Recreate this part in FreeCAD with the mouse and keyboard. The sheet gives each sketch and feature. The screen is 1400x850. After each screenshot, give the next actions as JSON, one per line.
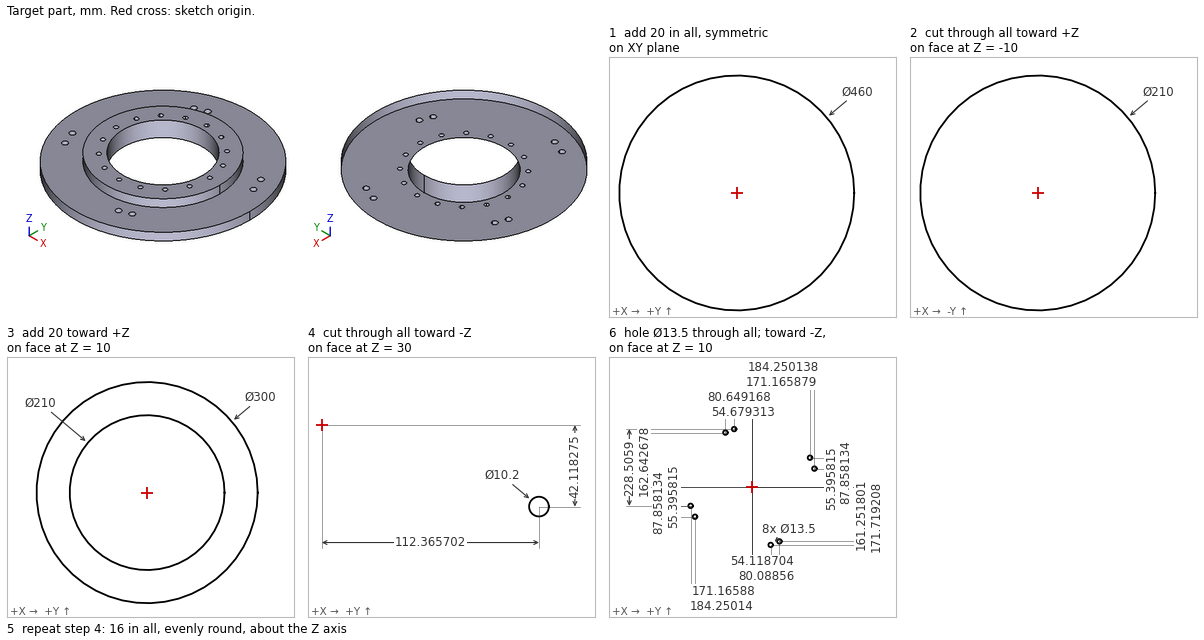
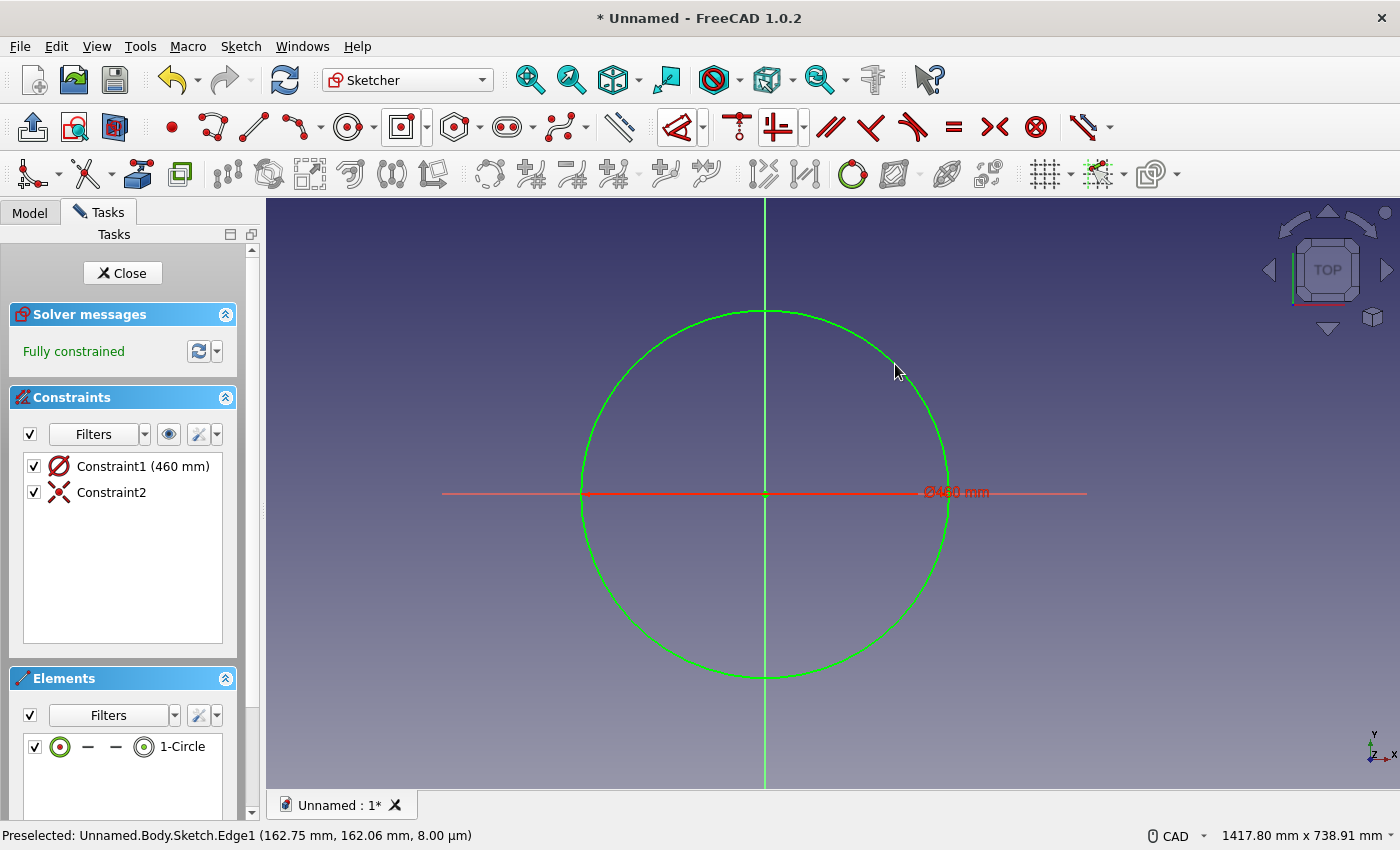
{"action": "left_click", "coordinate": [123, 273]}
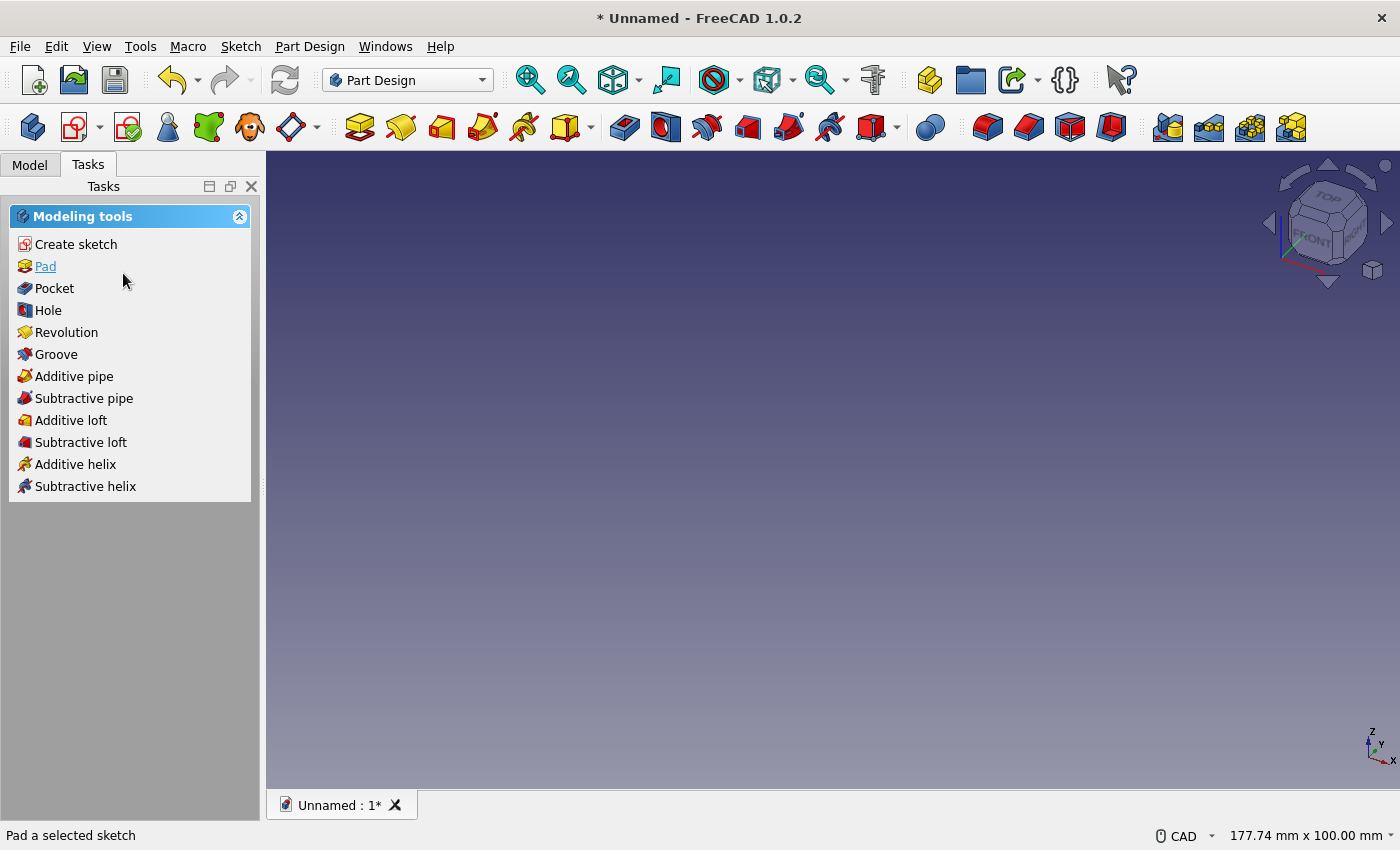
{"action": "left_click", "coordinate": [360, 128]}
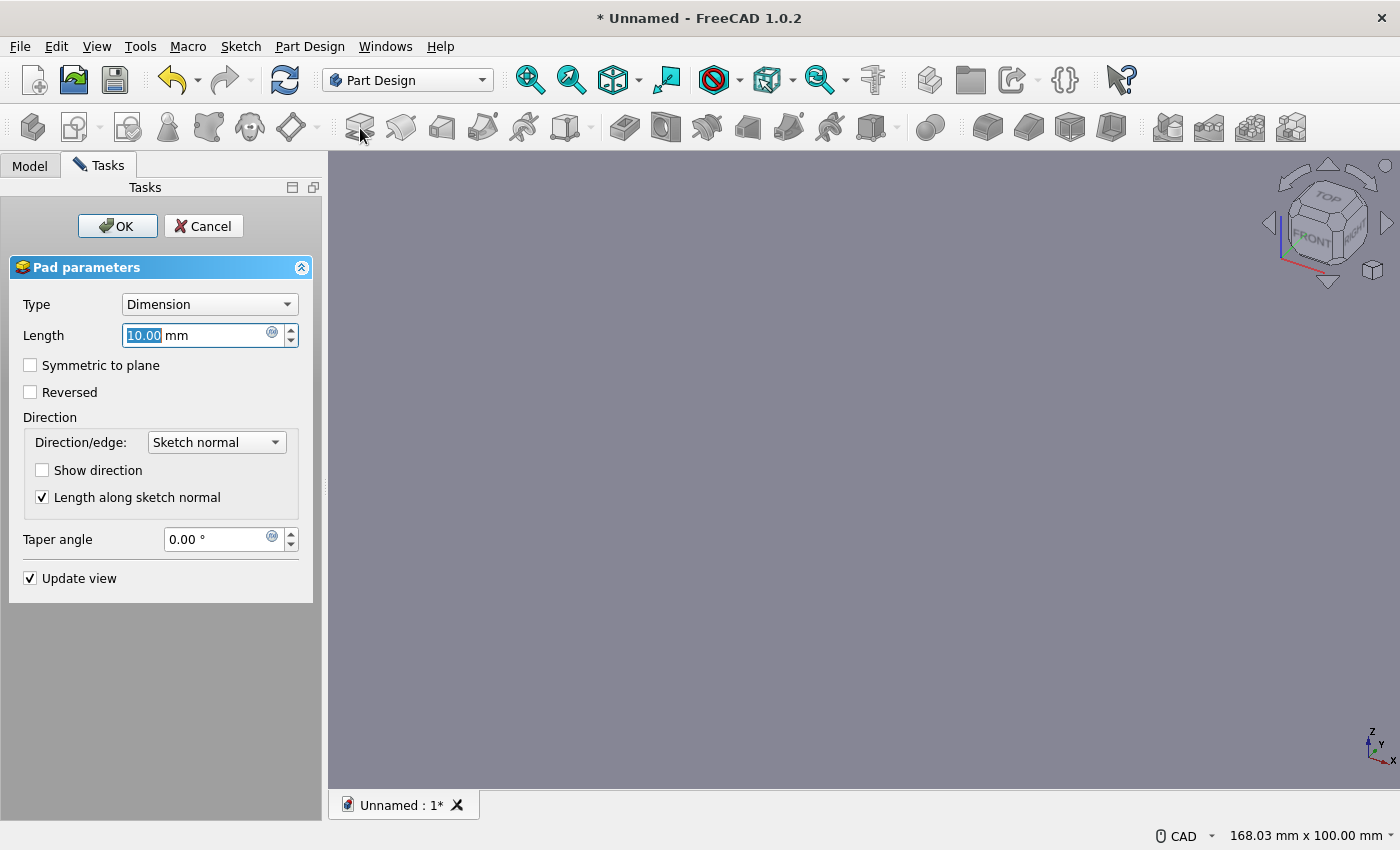
{"action": "type", "text": "20"}
{"action": "key", "text": "Tab"}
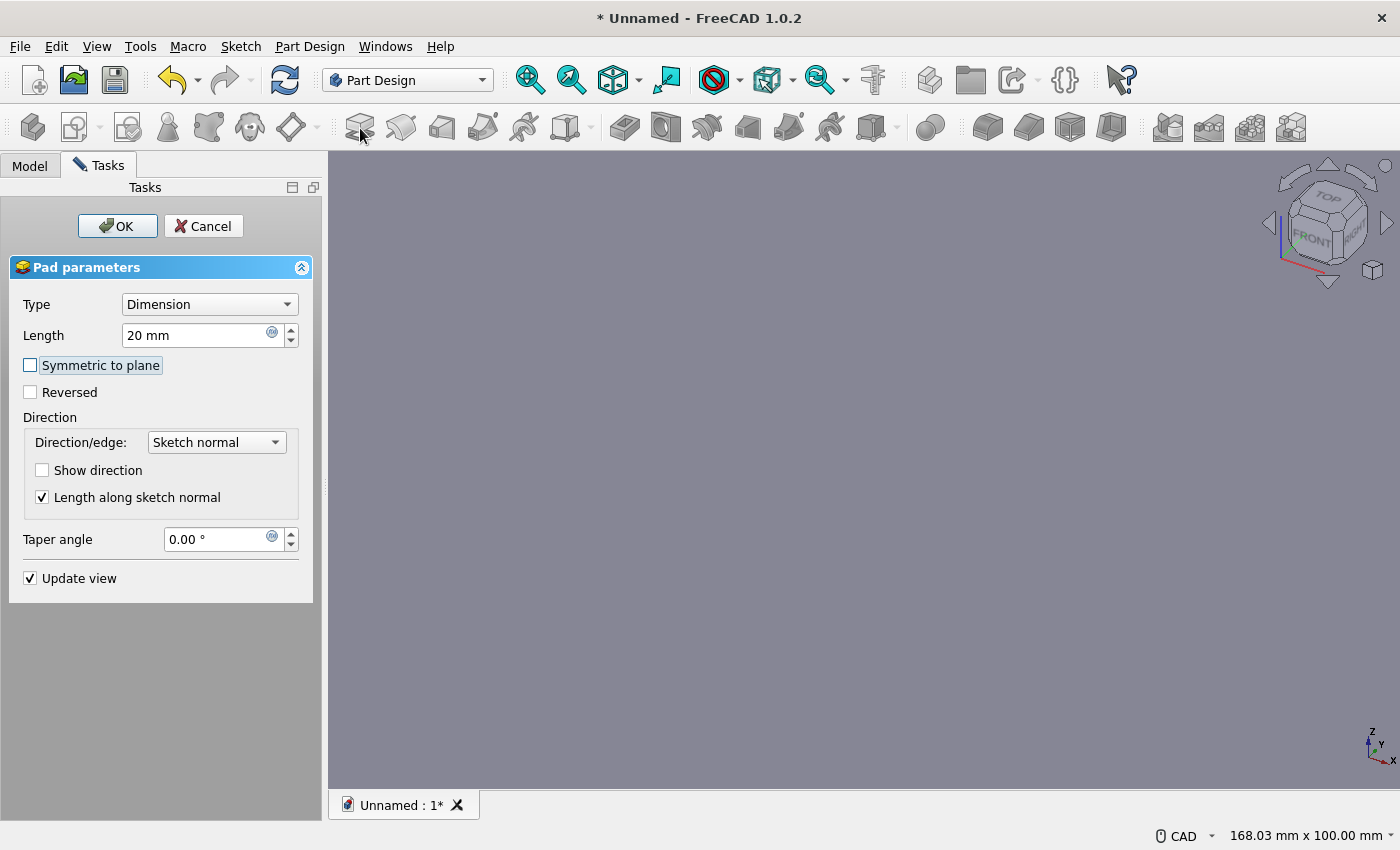
{"action": "left_click", "coordinate": [31, 365]}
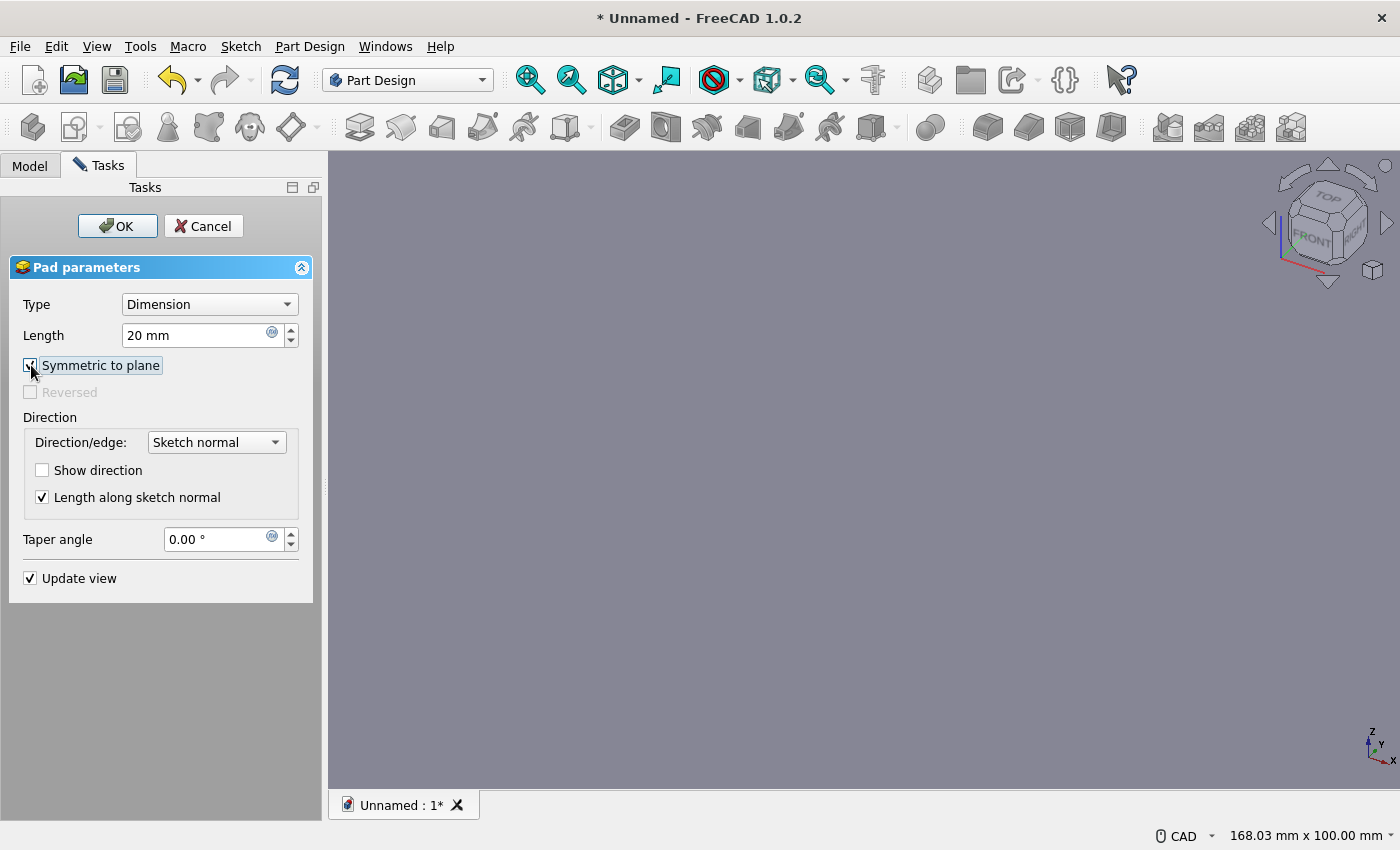
{"action": "left_click", "coordinate": [118, 226]}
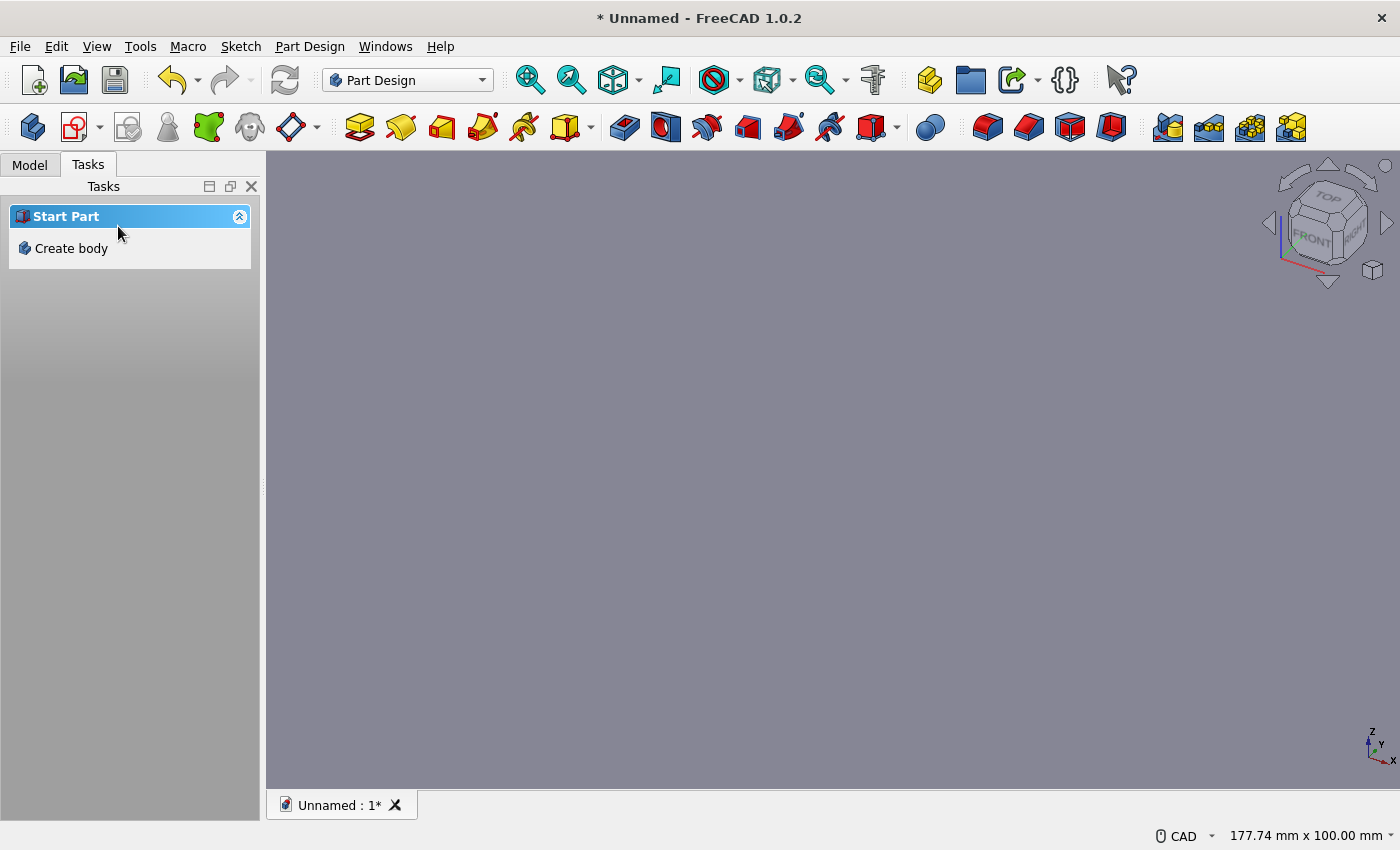
{"action": "left_click", "coordinate": [531, 80]}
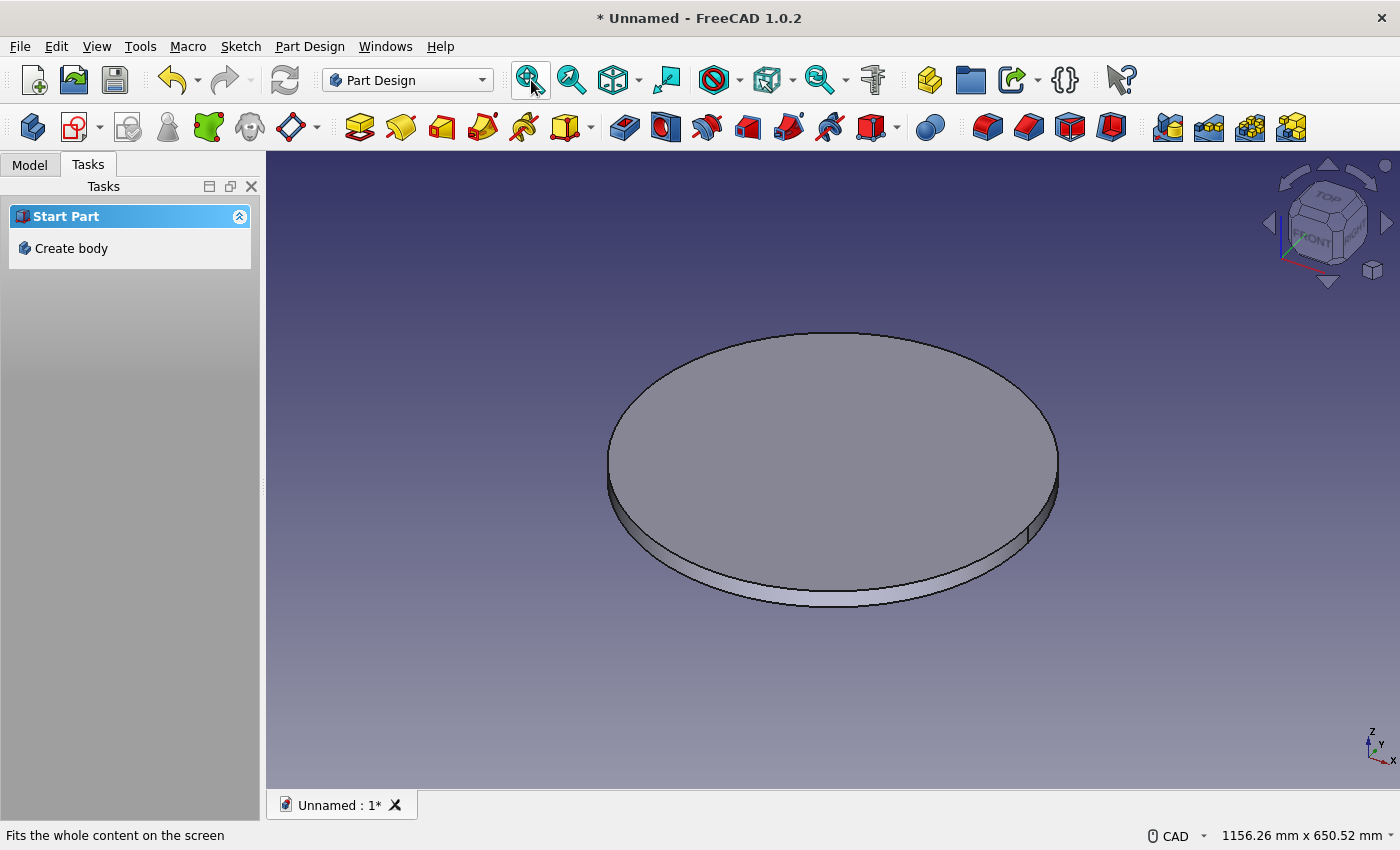
{"action": "key", "text": "5"}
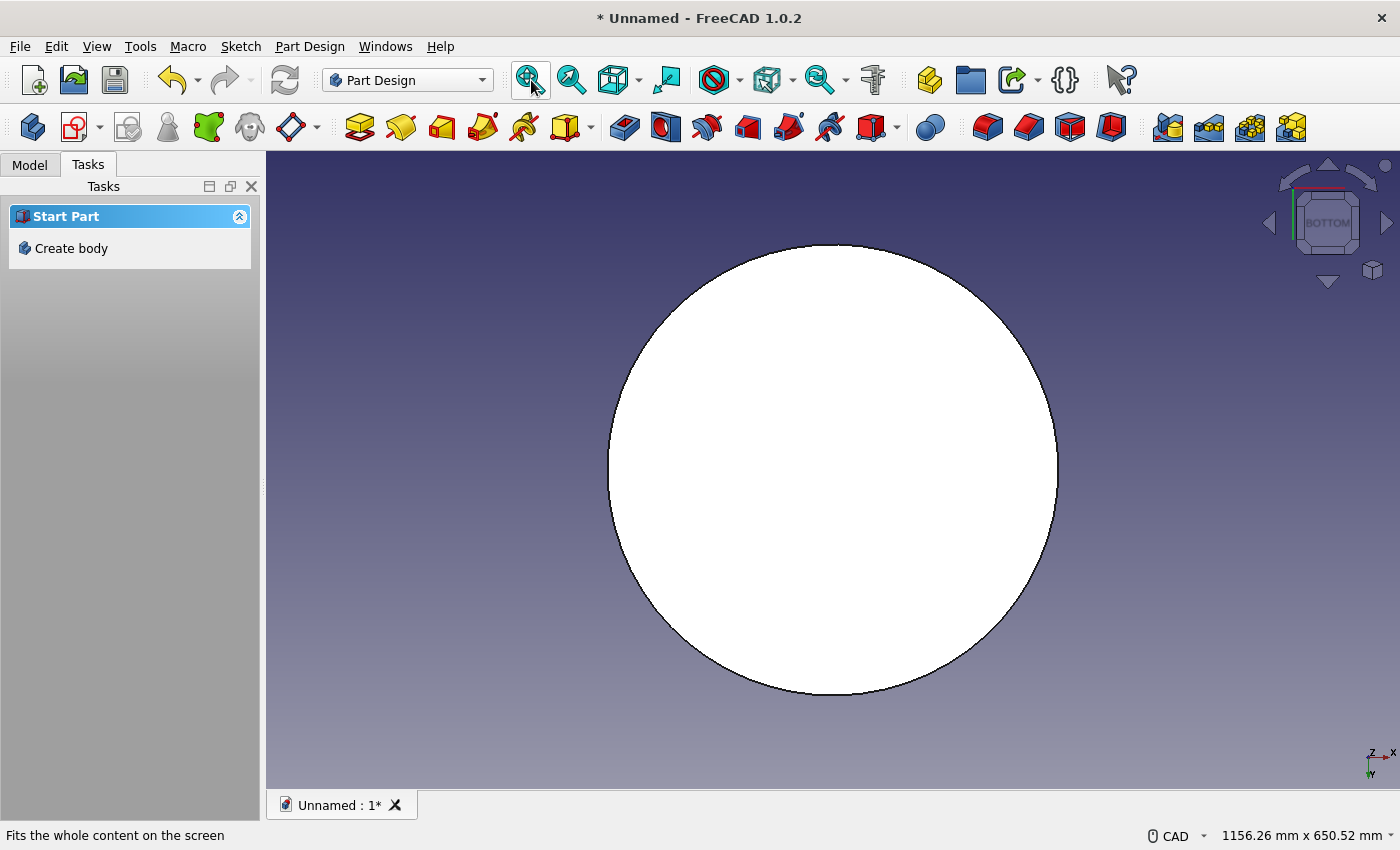
{"action": "left_click", "coordinate": [833, 469]}